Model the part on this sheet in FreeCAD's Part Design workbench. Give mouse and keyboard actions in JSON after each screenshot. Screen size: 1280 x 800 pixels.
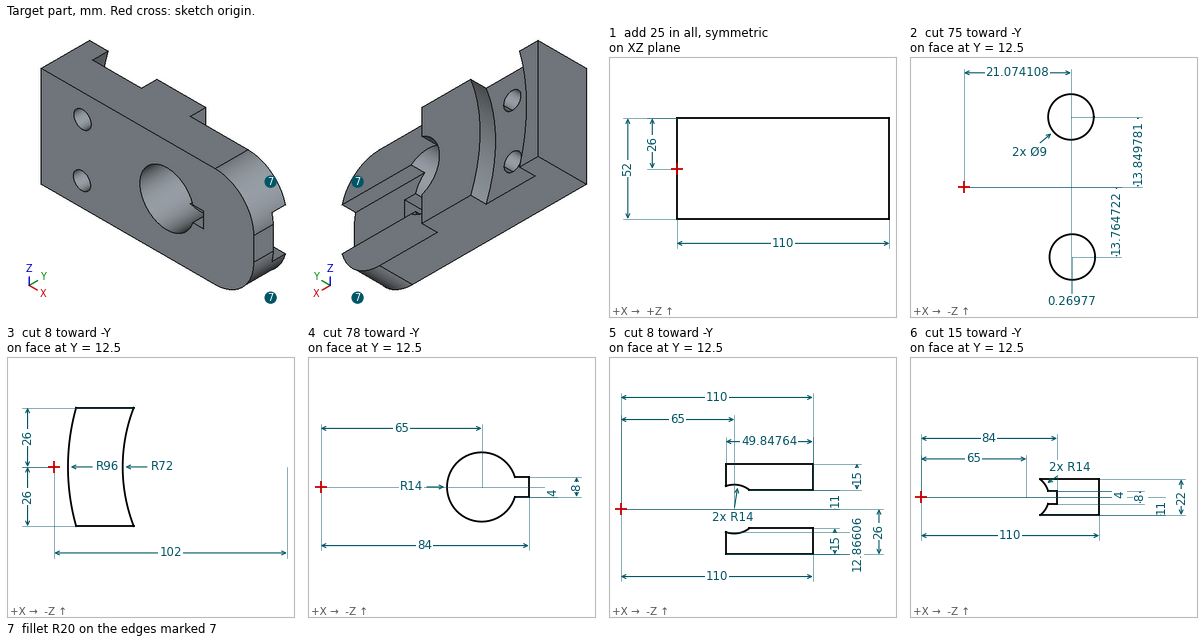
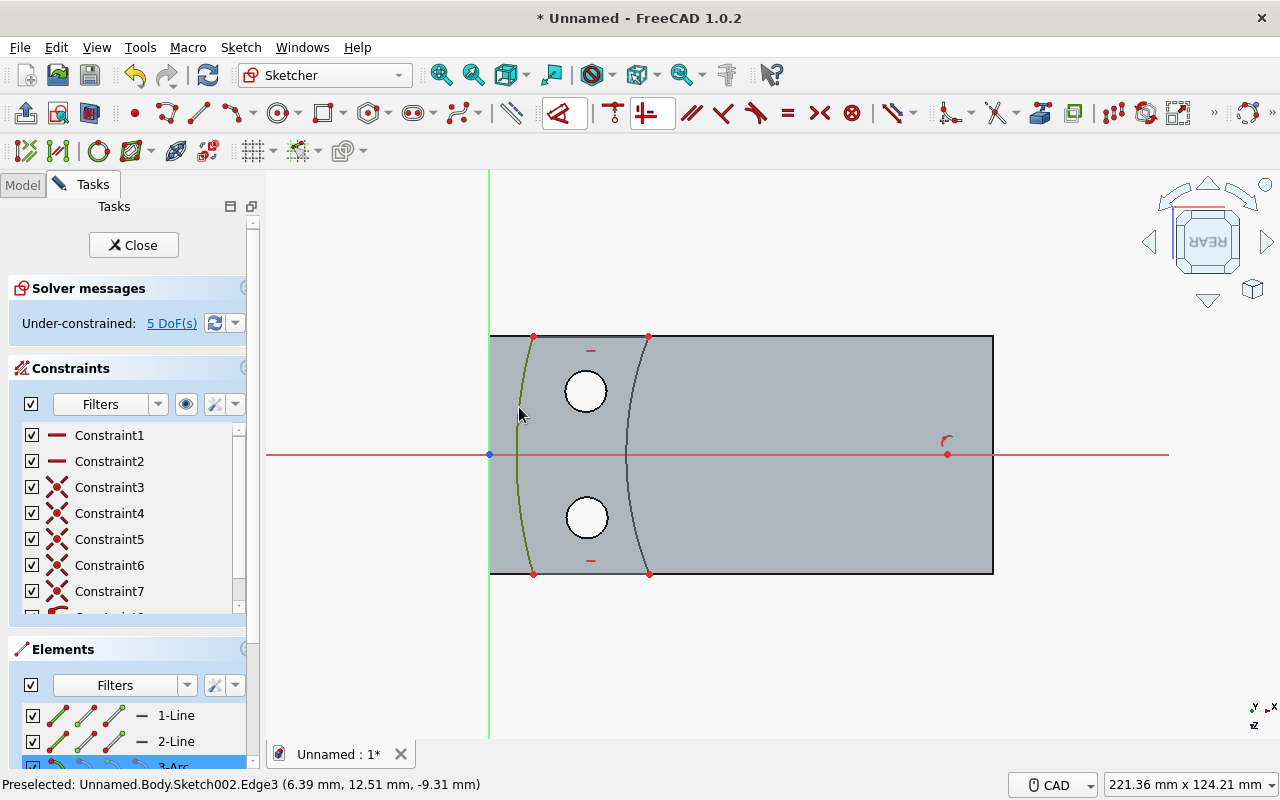
{"action": "key", "text": "k r"}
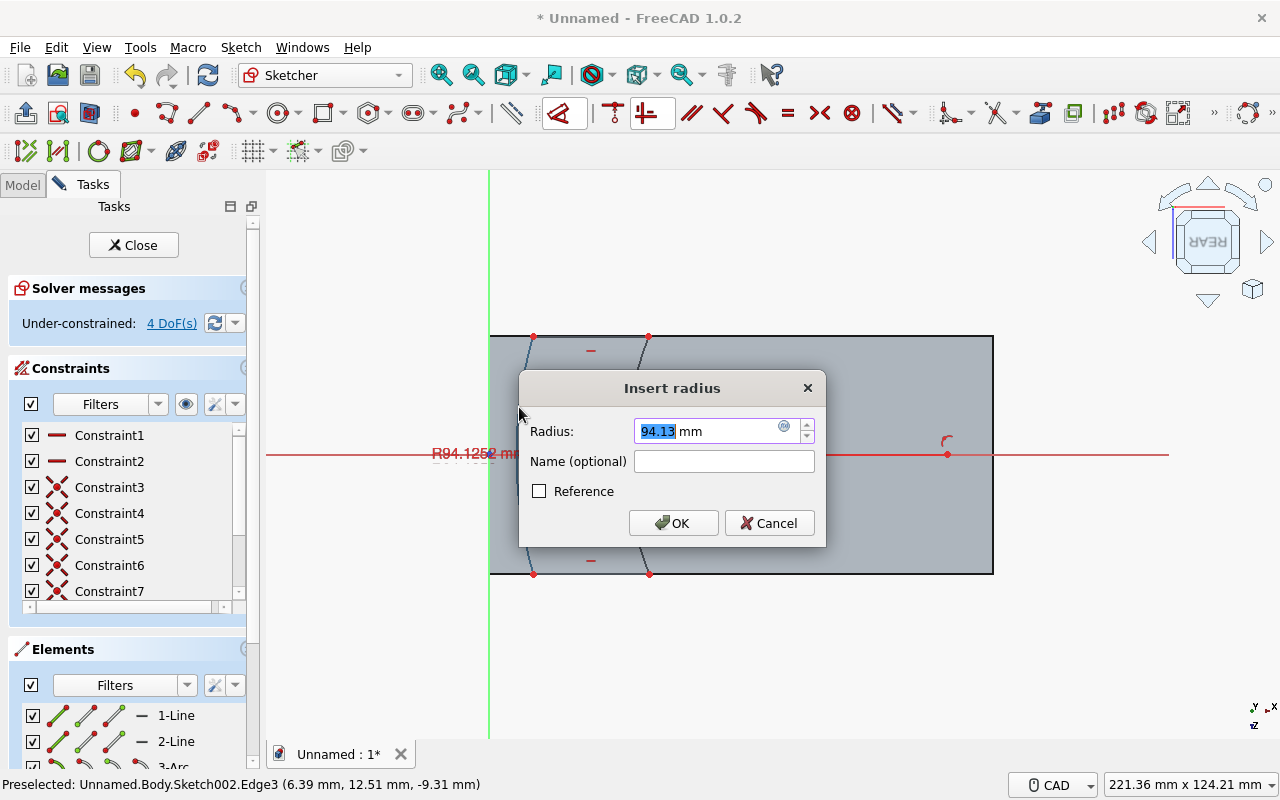
{"action": "type", "text": "96"}
{"action": "key", "text": "Return"}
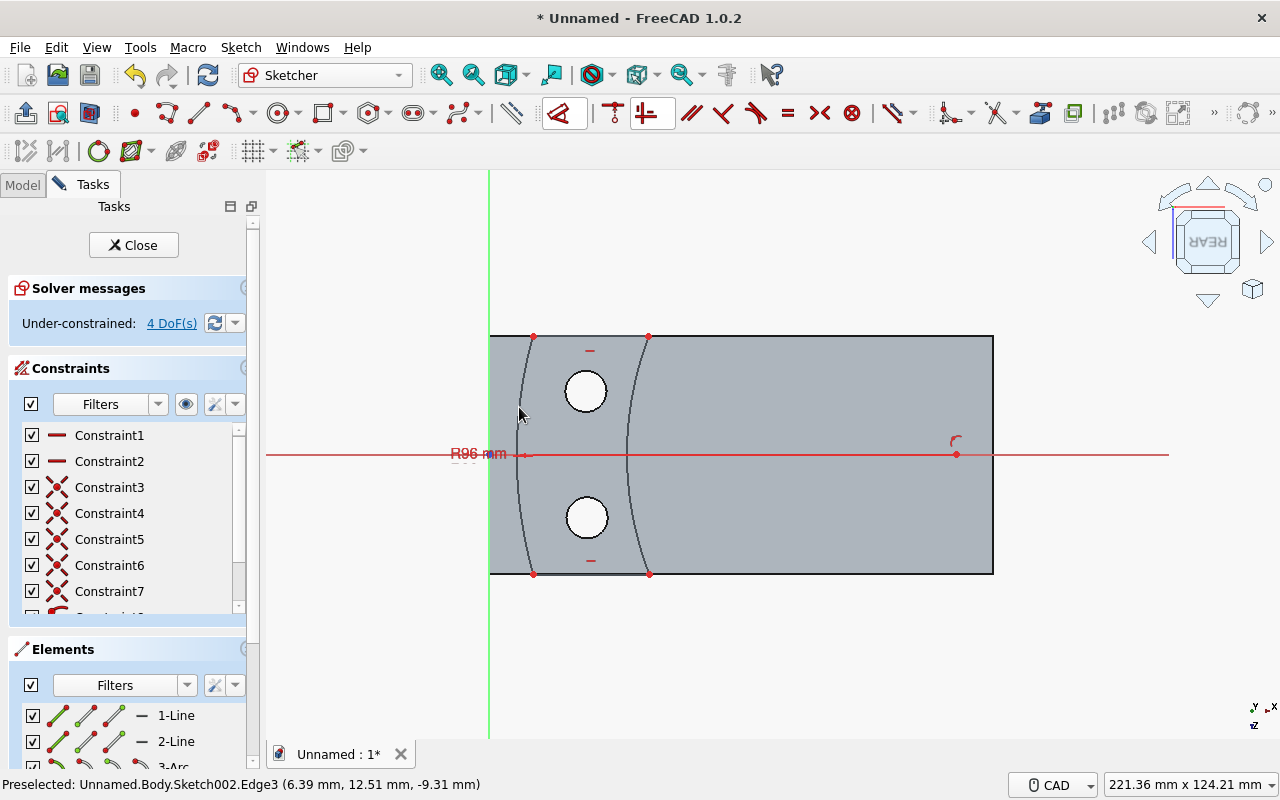
{"action": "left_click", "coordinate": [630, 407]}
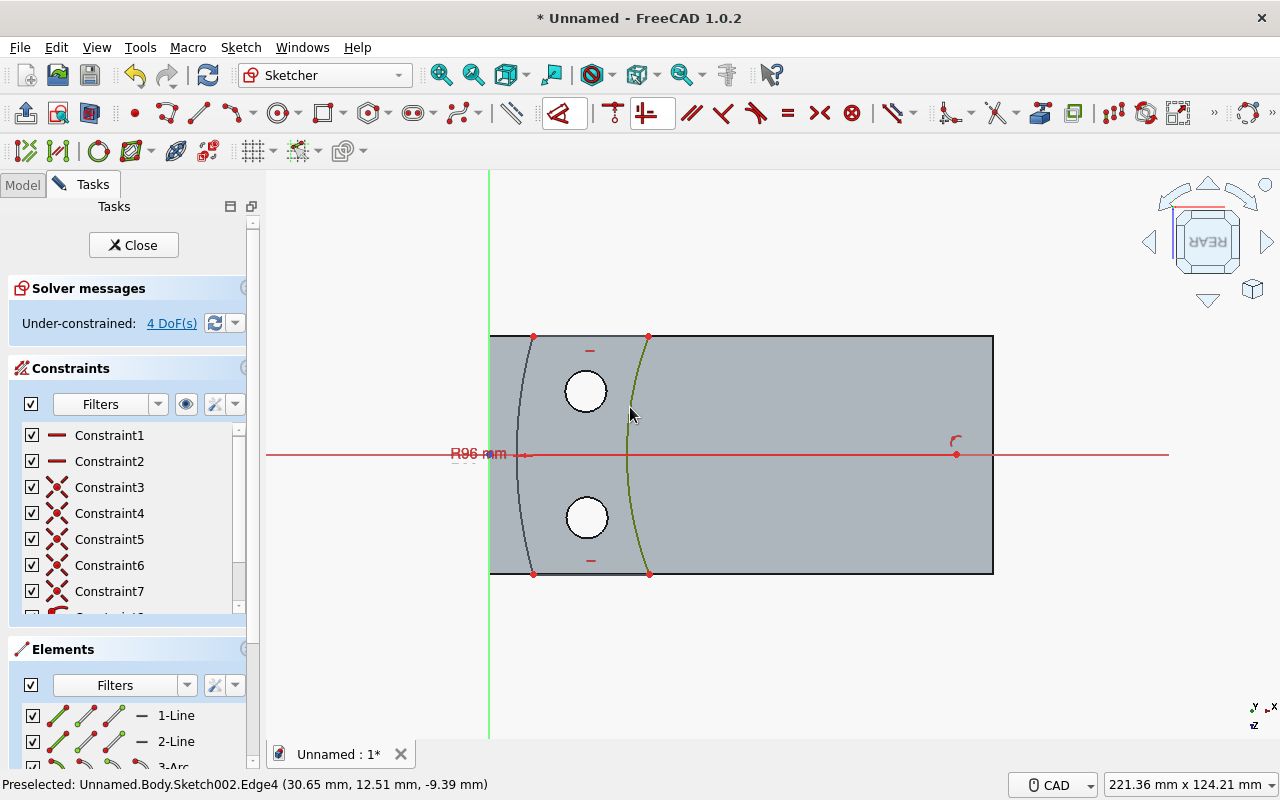
{"action": "left_click", "coordinate": [582, 114]}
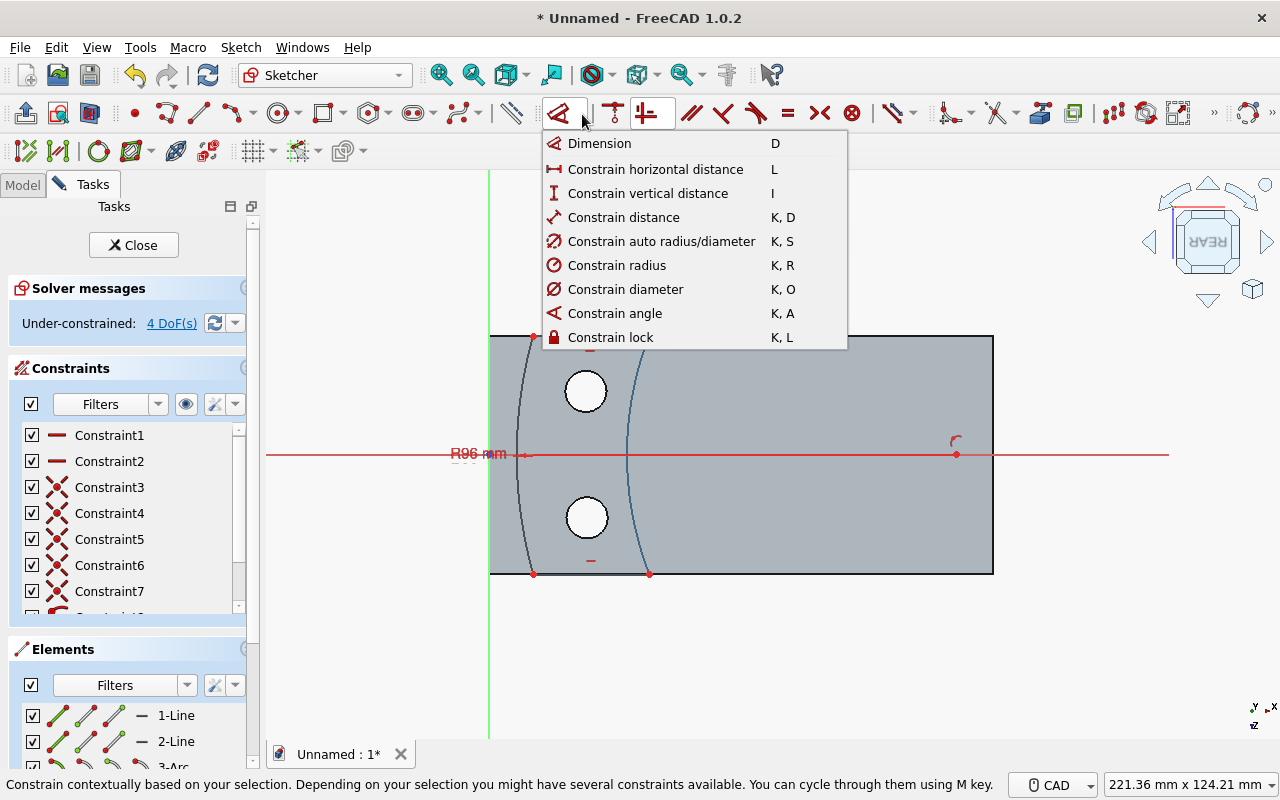
{"action": "left_click", "coordinate": [695, 265]}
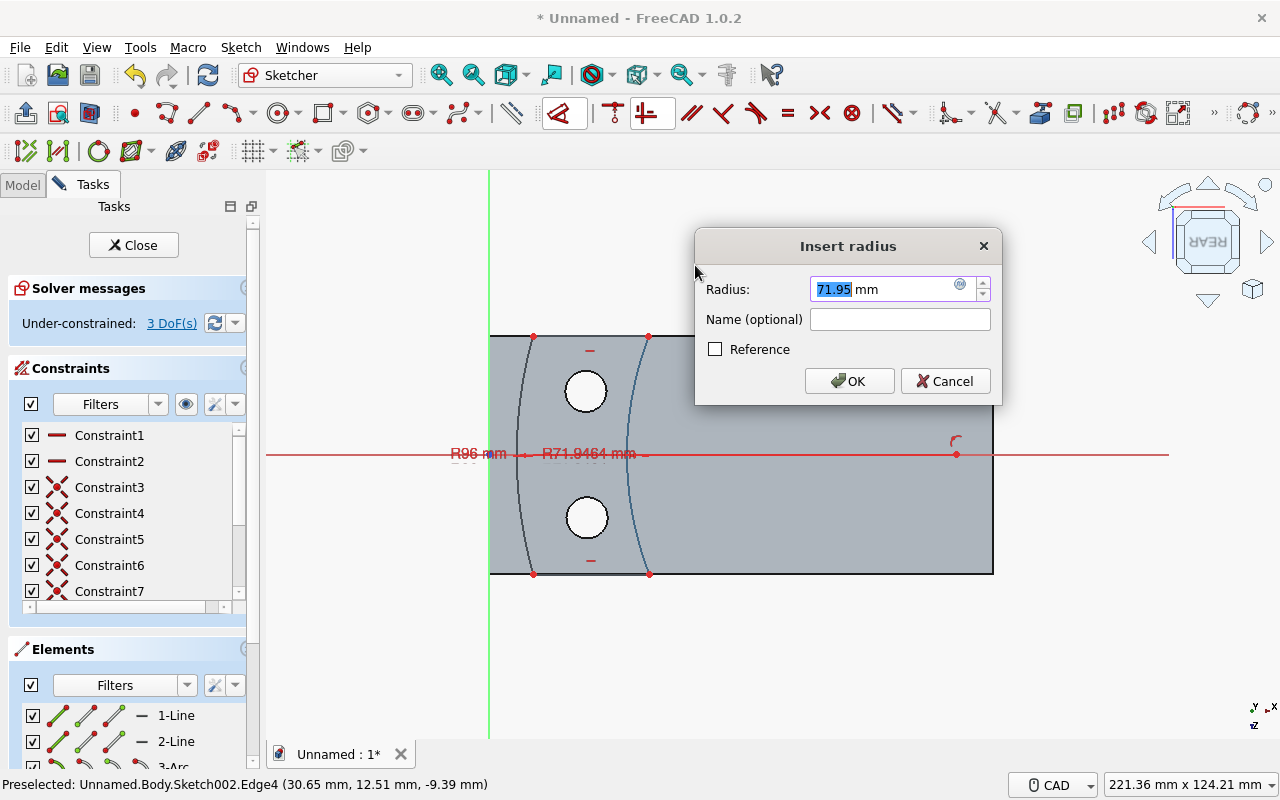
{"action": "type", "text": "72"}
{"action": "key", "text": "Return"}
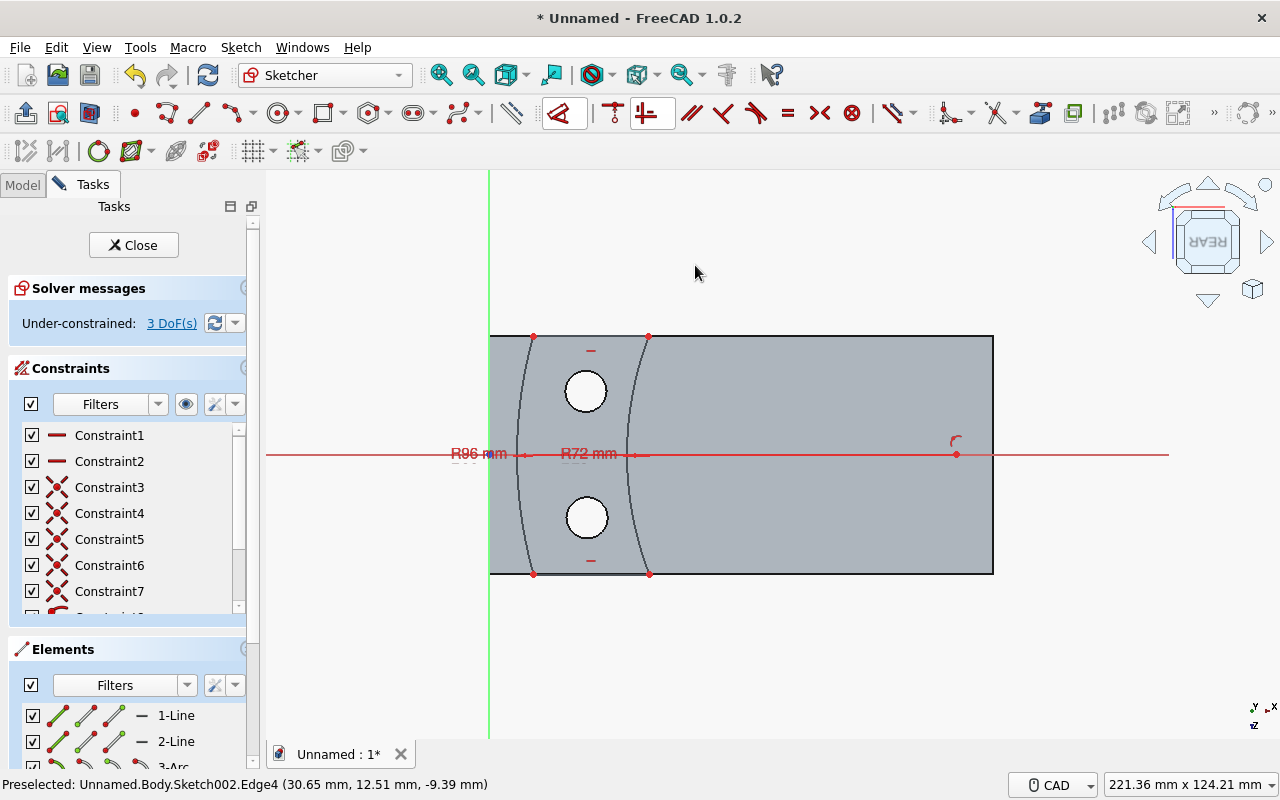
{"action": "left_click", "coordinate": [649, 336]}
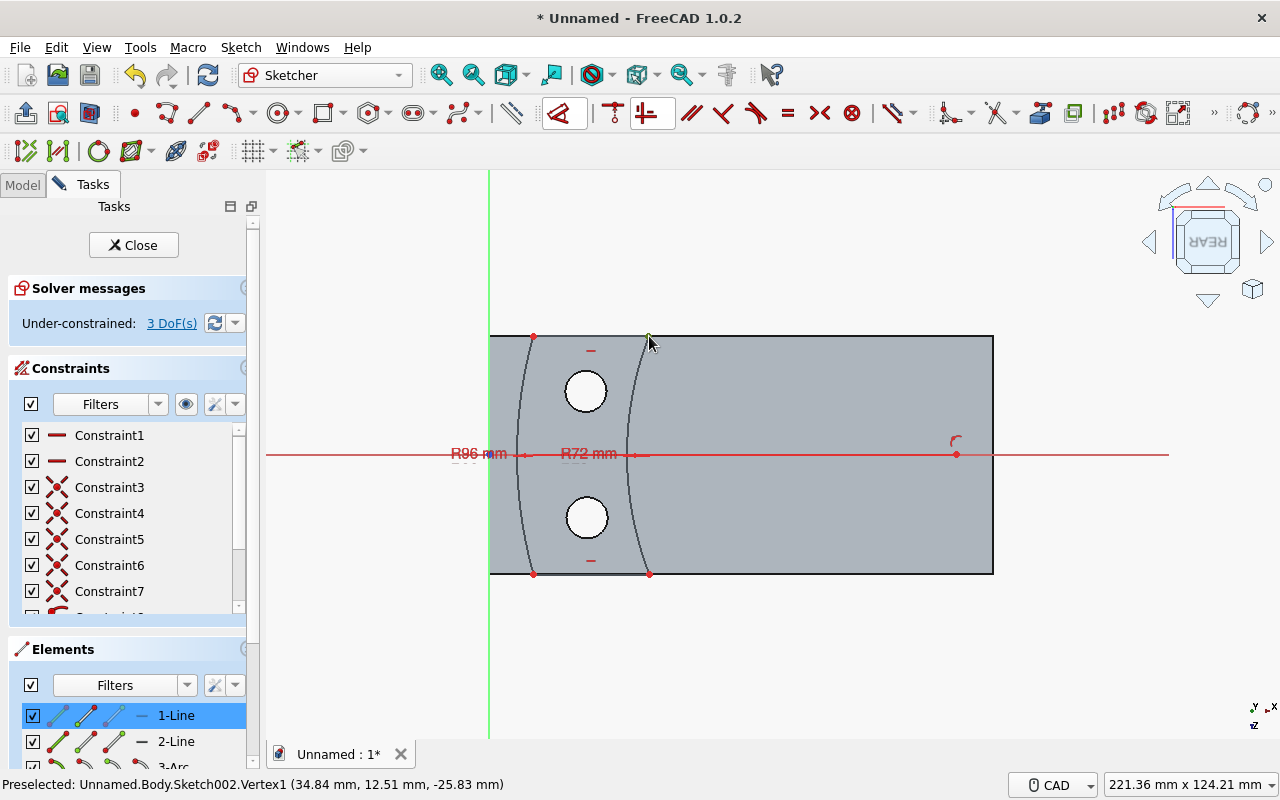
{"action": "left_click", "coordinate": [582, 114]}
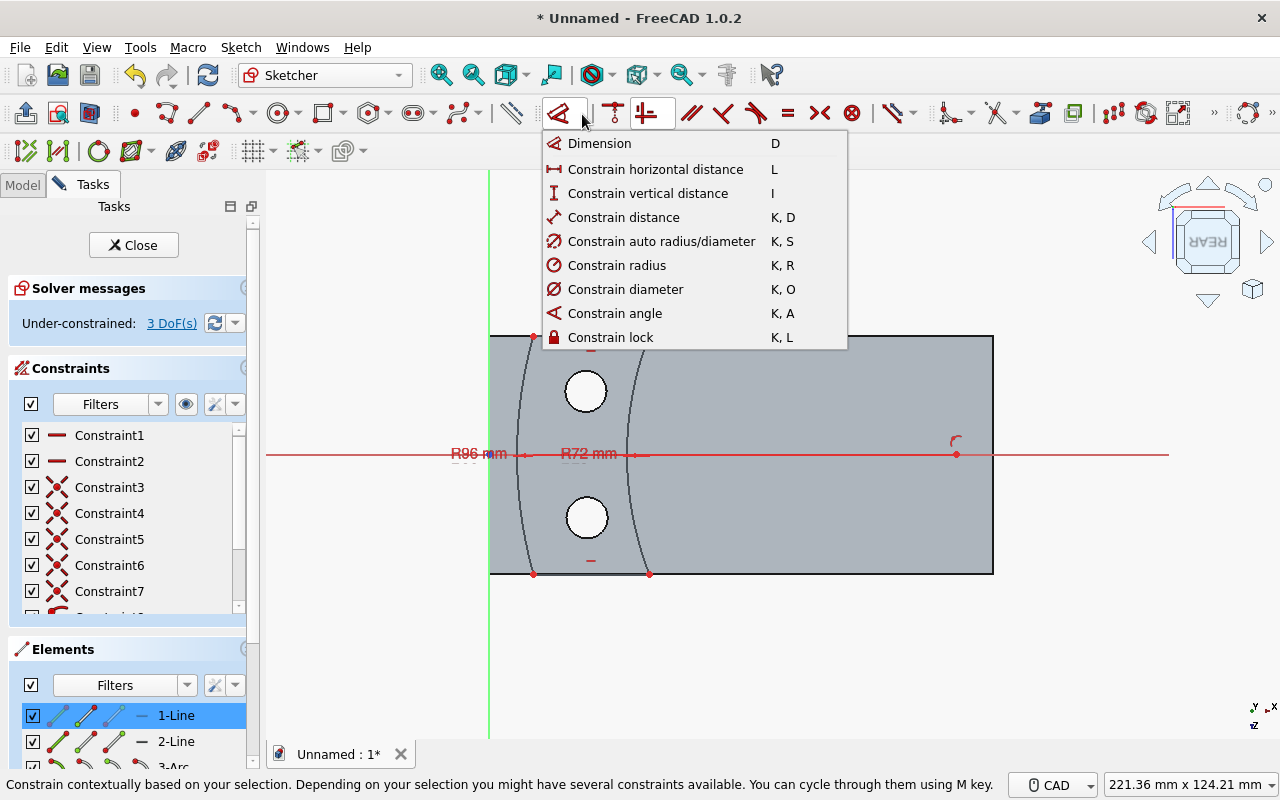
{"action": "left_click", "coordinate": [695, 193]}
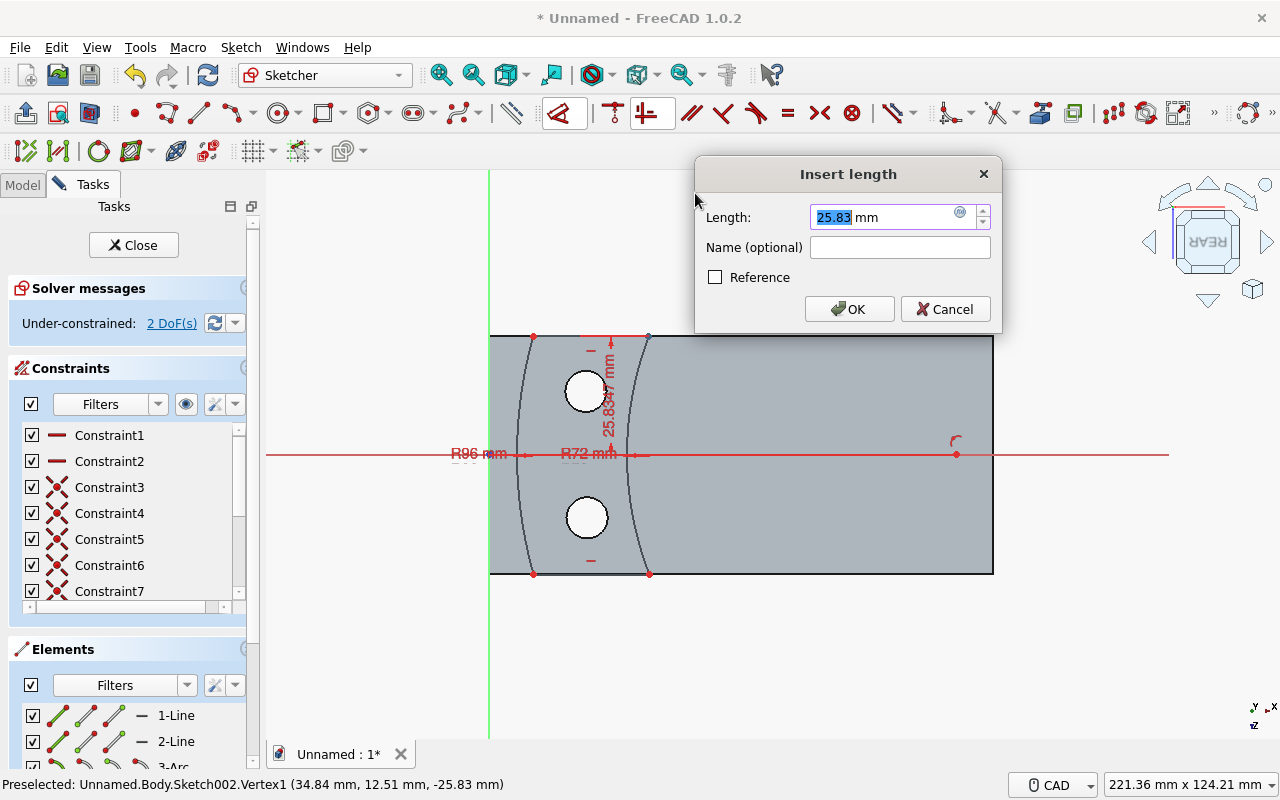
{"action": "type", "text": "26"}
{"action": "key", "text": "Return"}